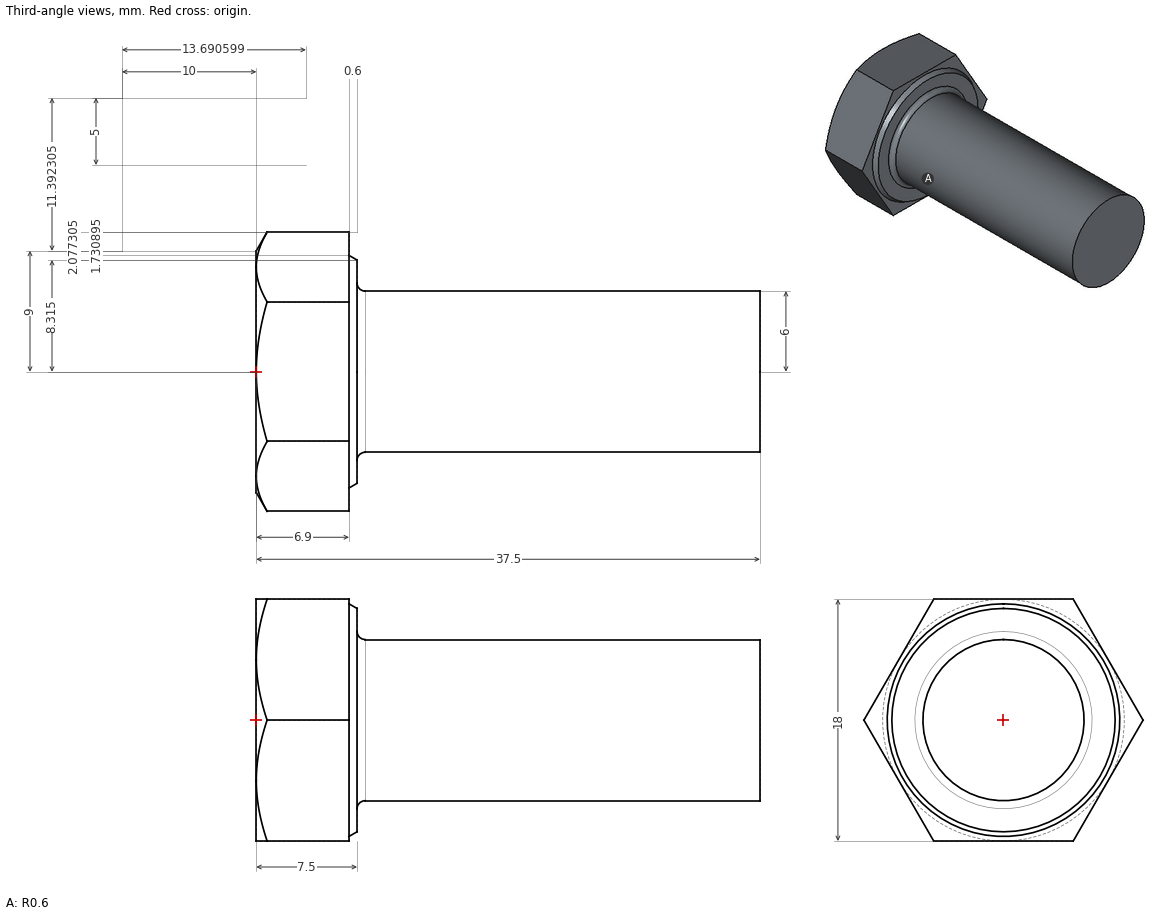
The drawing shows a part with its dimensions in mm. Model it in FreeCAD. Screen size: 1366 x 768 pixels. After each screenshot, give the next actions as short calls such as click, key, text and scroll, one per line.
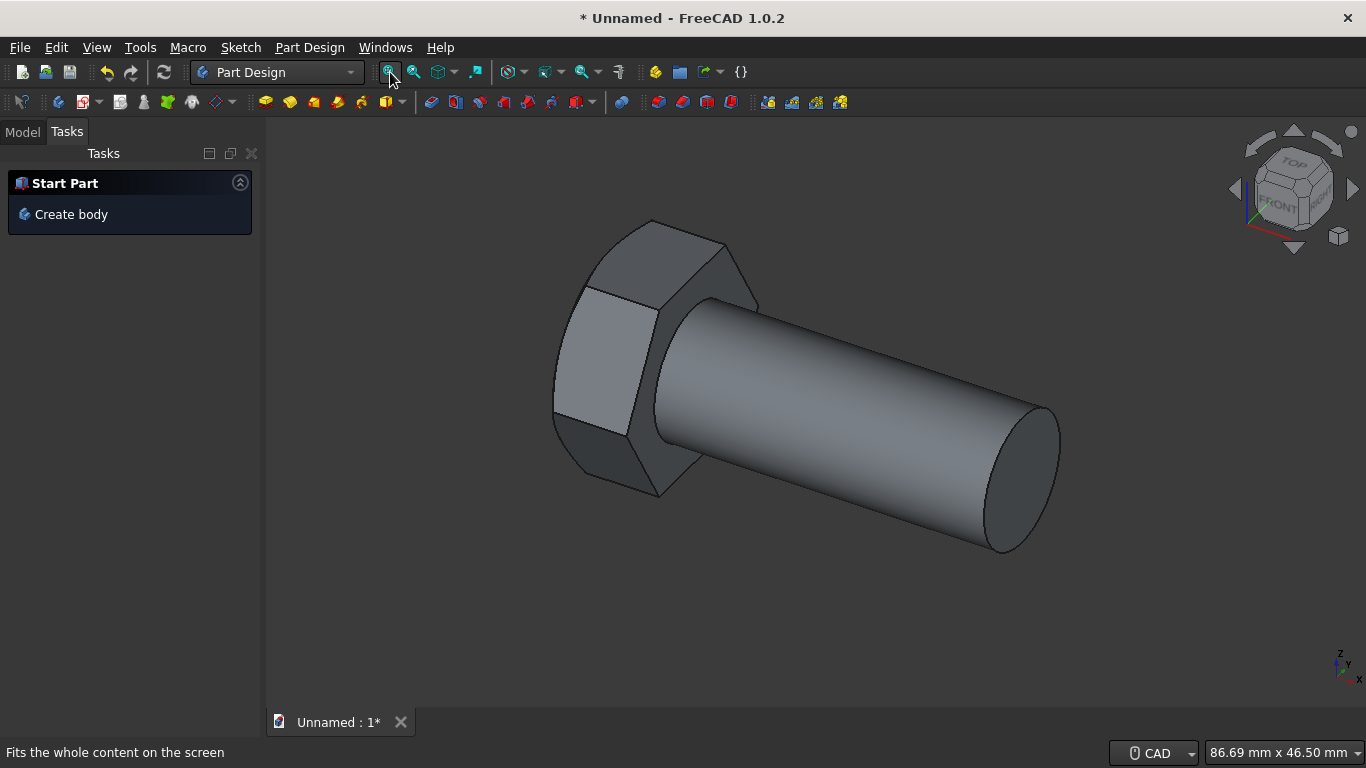
click(84, 102)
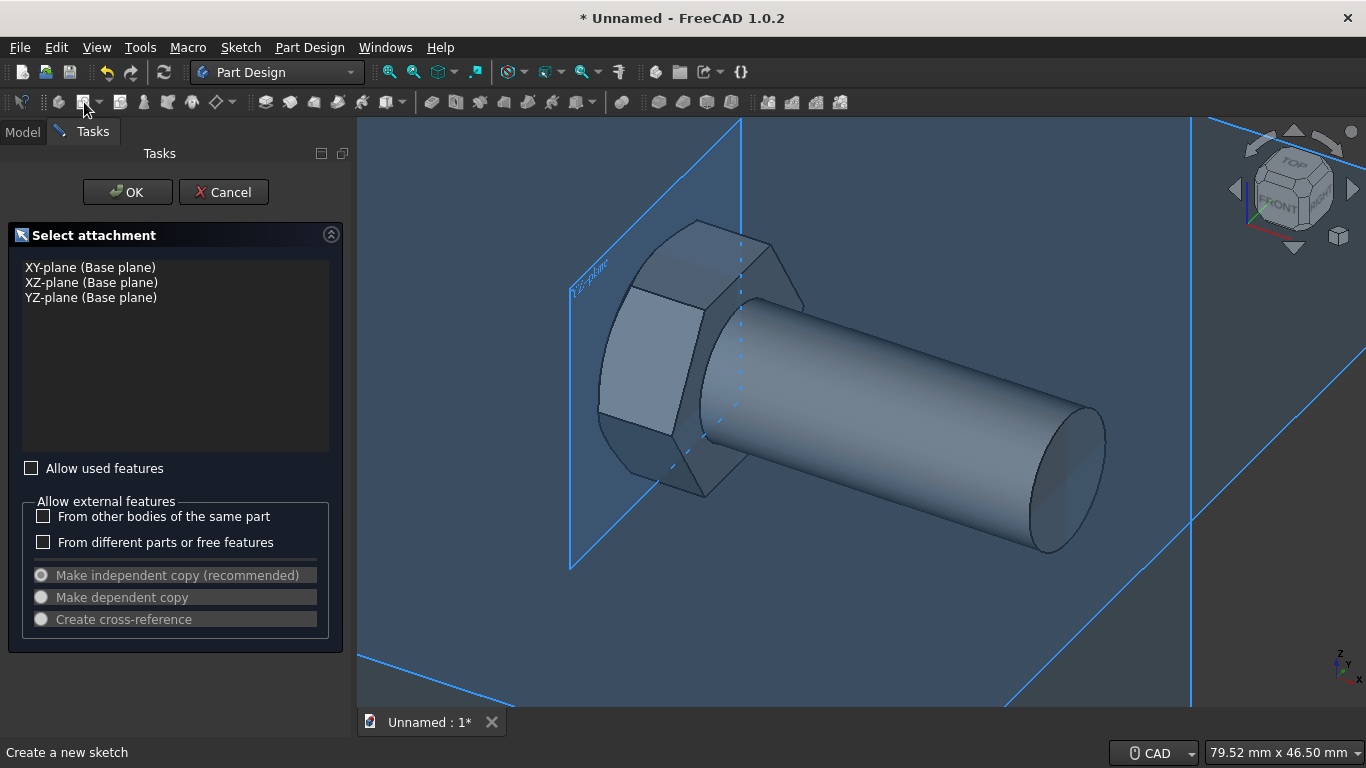
click(82, 268)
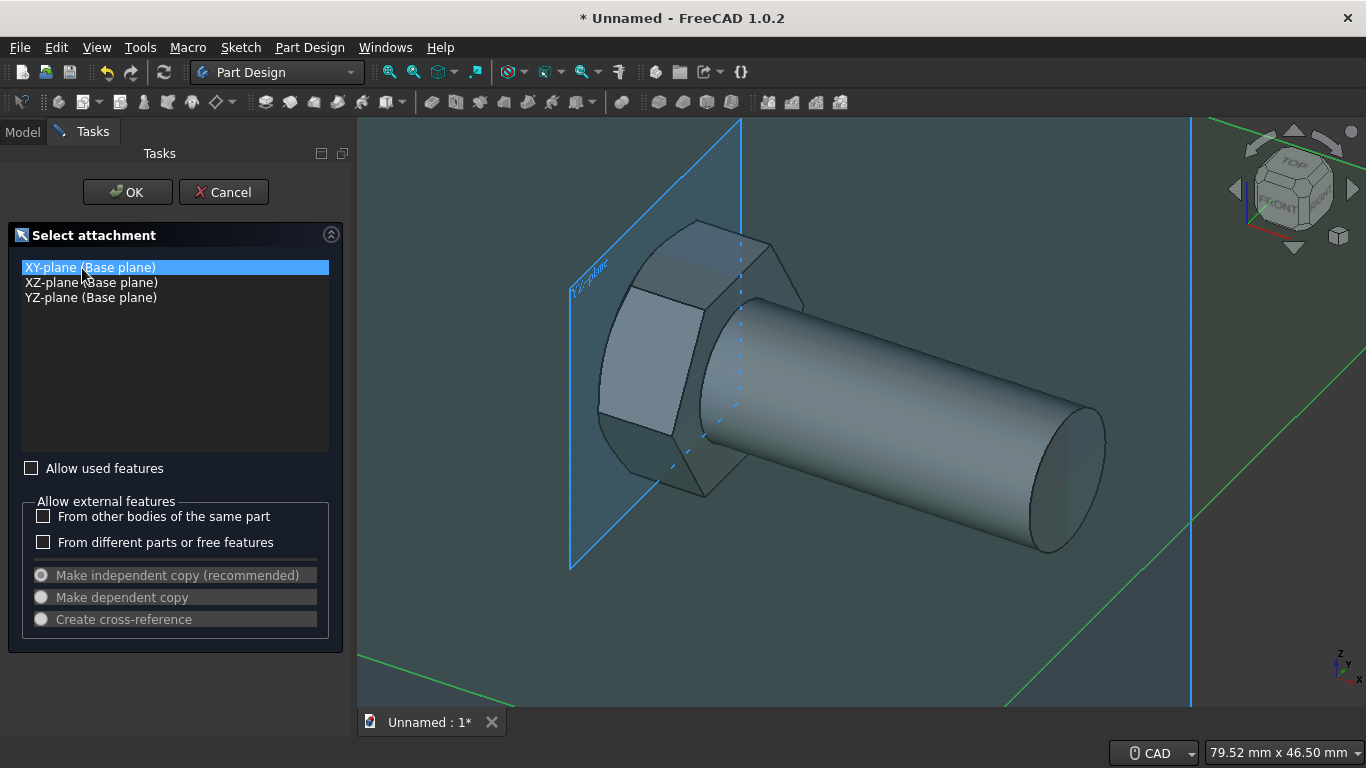
click(128, 192)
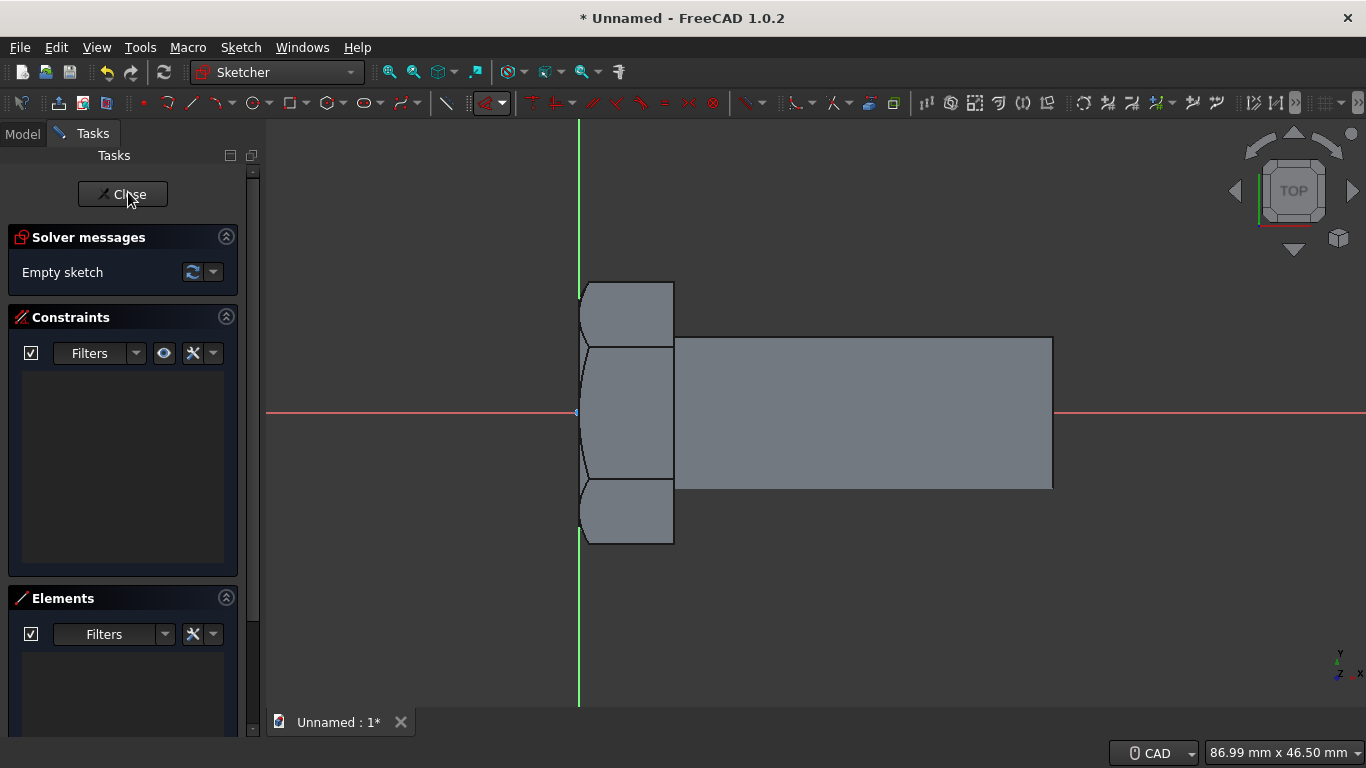
key(q)
key(s)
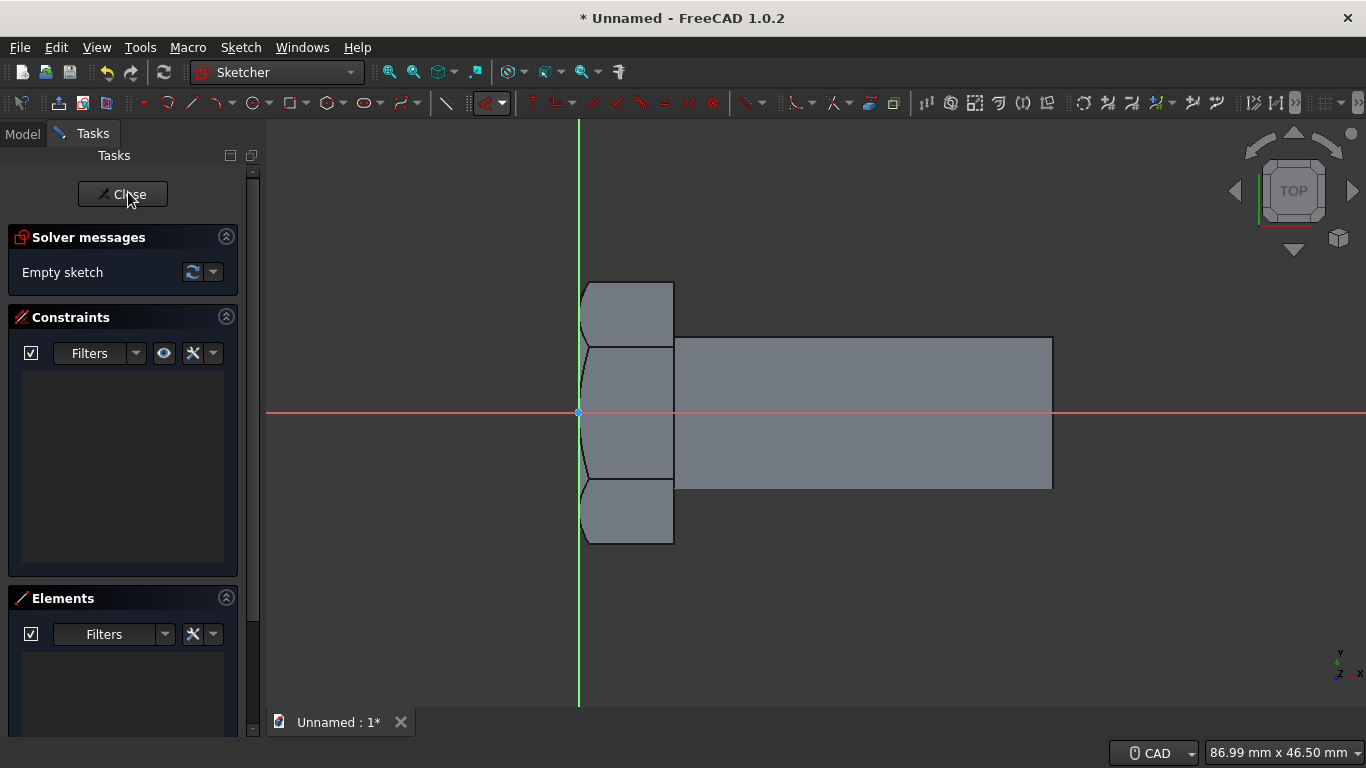
scroll(664, 285, up, 13)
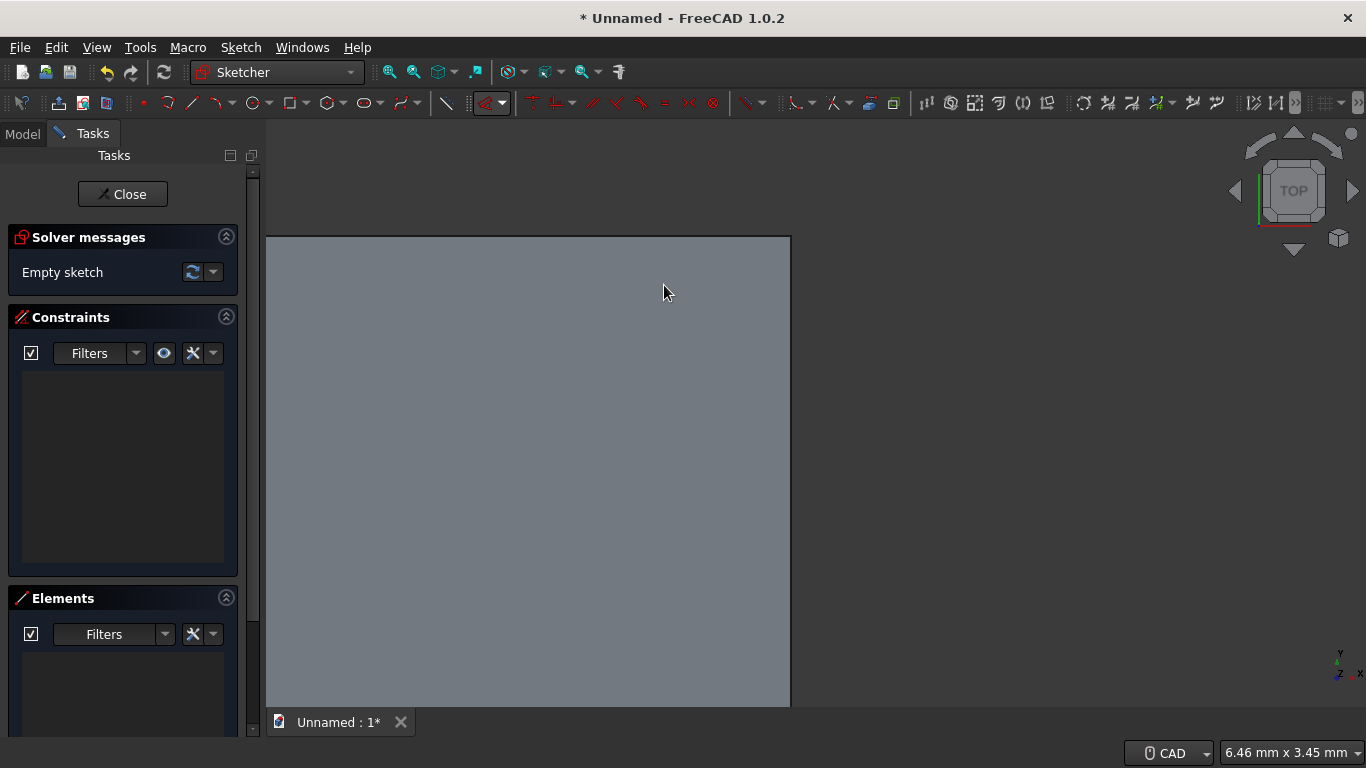
key(g)
key(m)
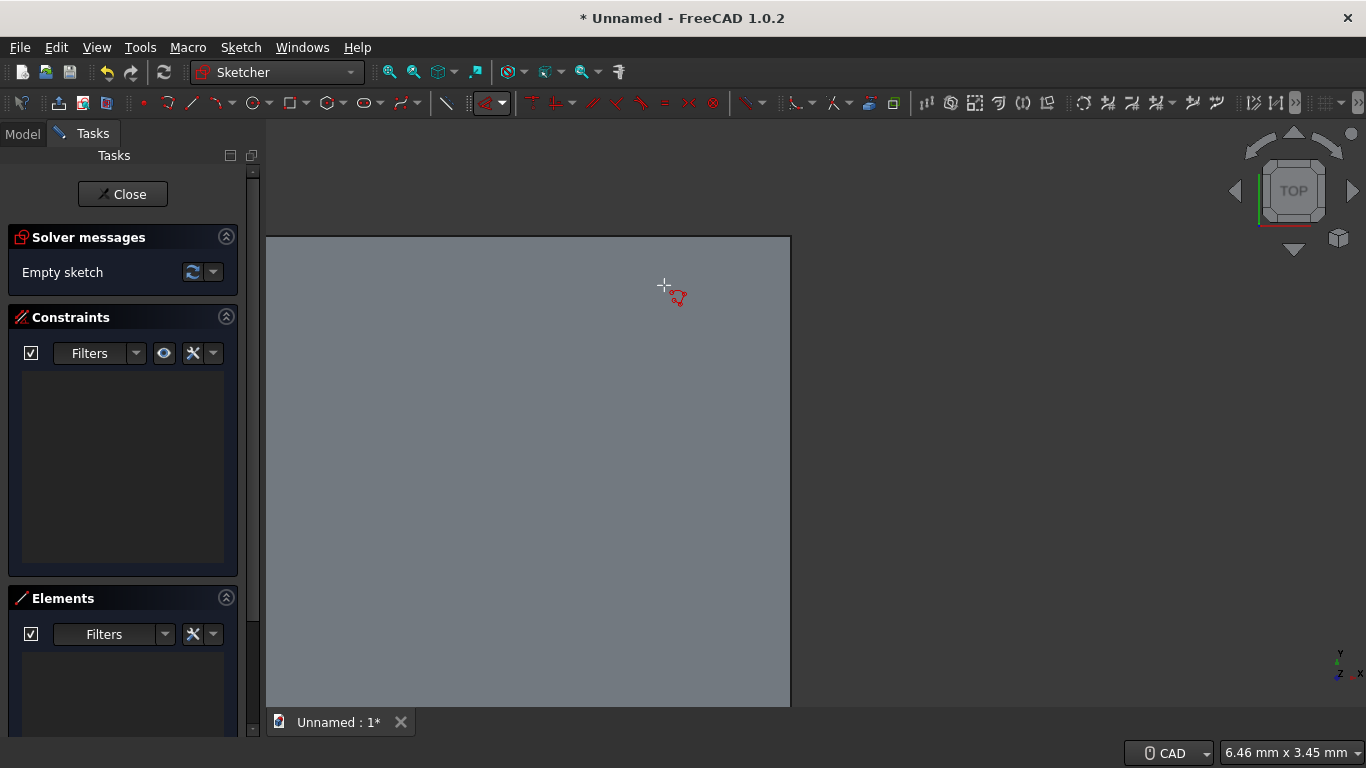
click(688, 530)
click(791, 589)
click(791, 236)
click(688, 236)
click(688, 531)
key(Escape)
key(Escape)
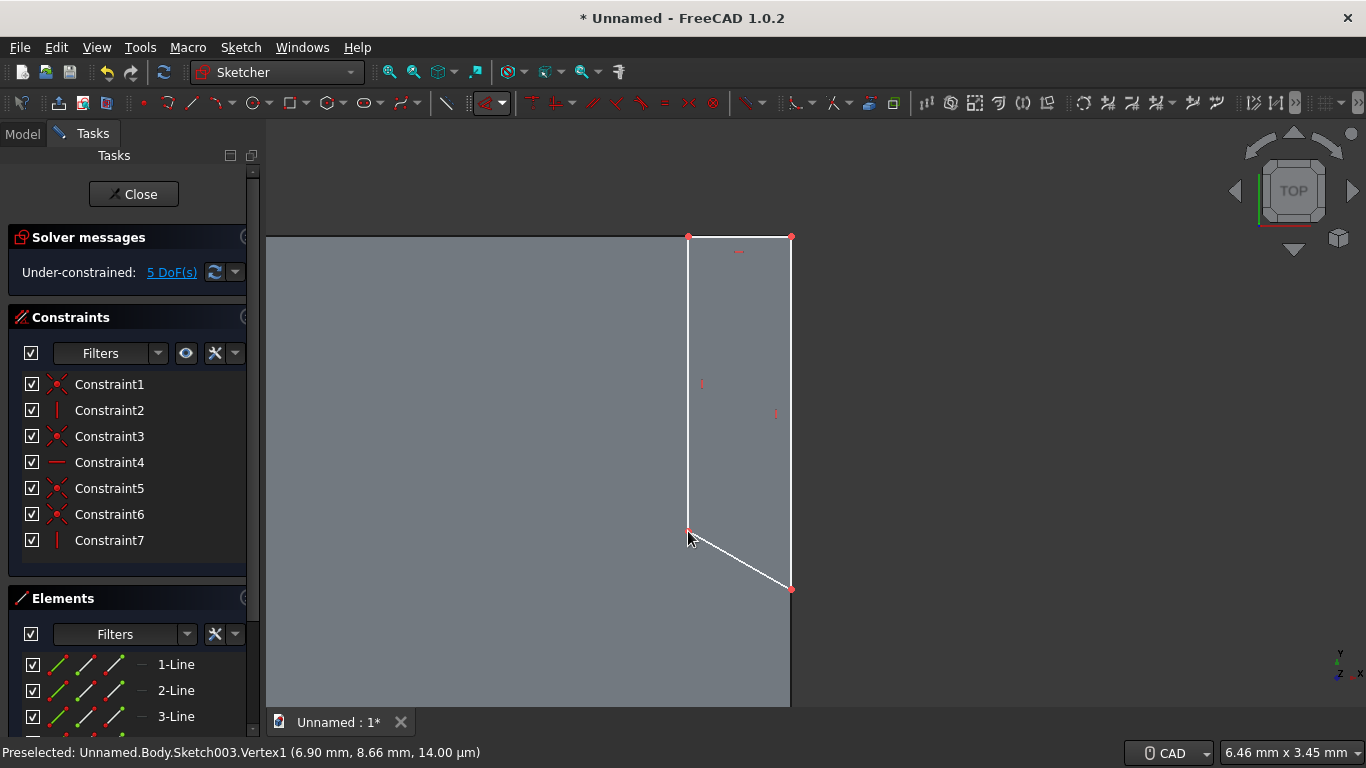
click(760, 237)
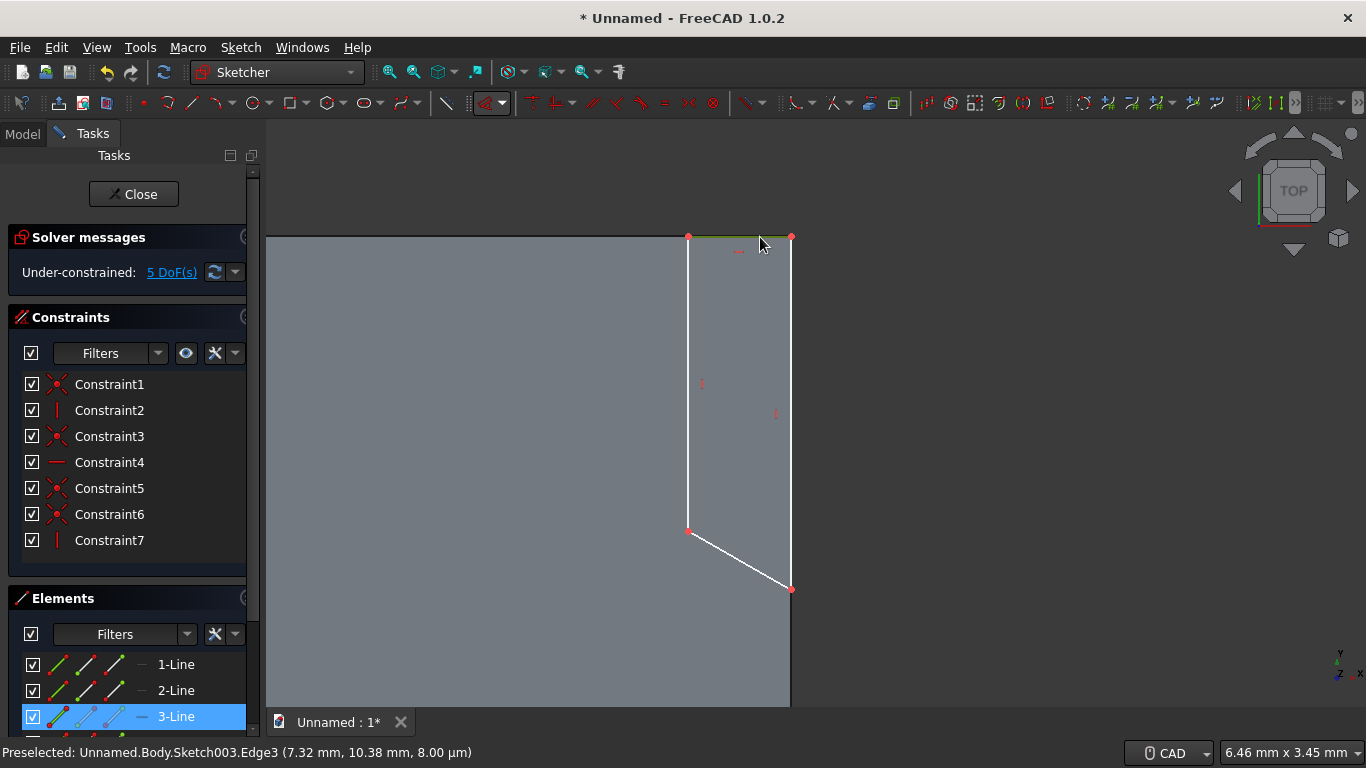
key(l)